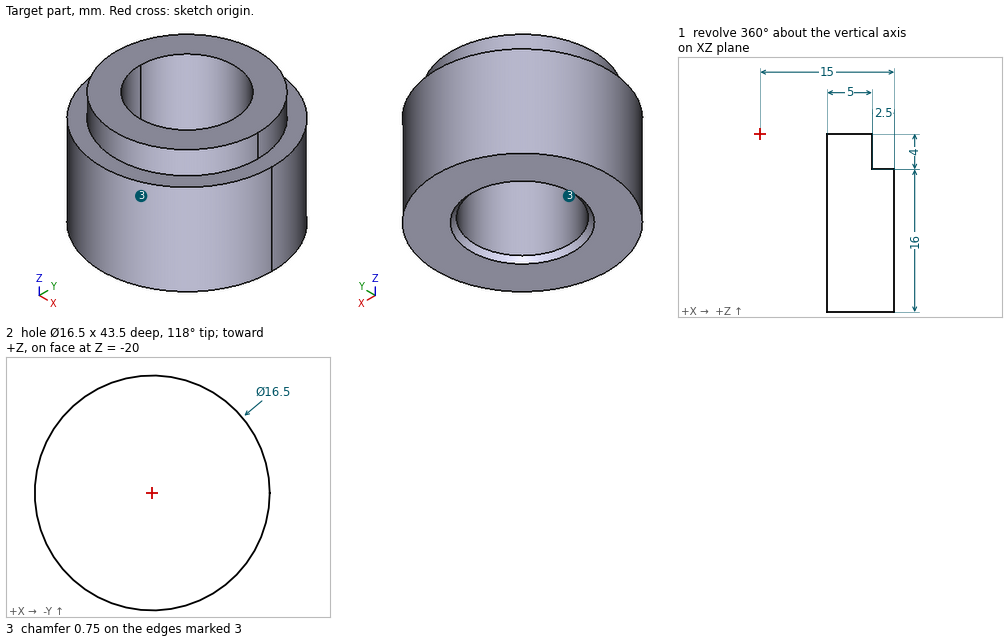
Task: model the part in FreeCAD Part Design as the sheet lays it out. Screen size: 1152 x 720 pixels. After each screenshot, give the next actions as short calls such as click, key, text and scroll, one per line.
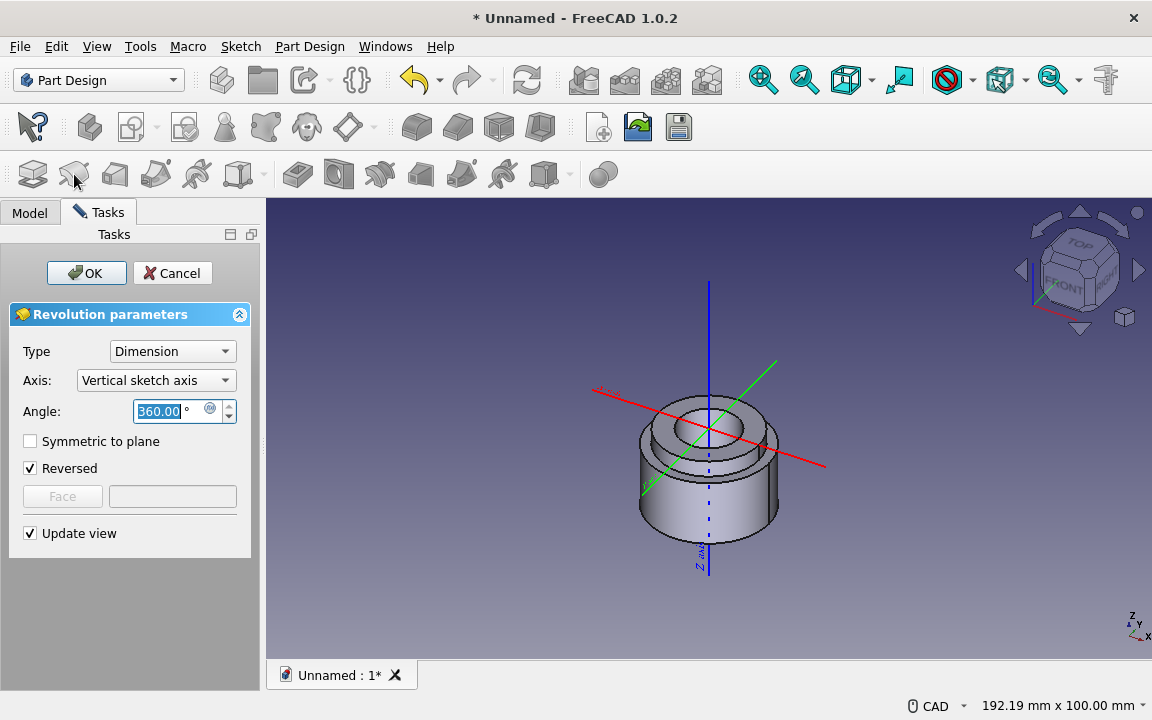
click(87, 273)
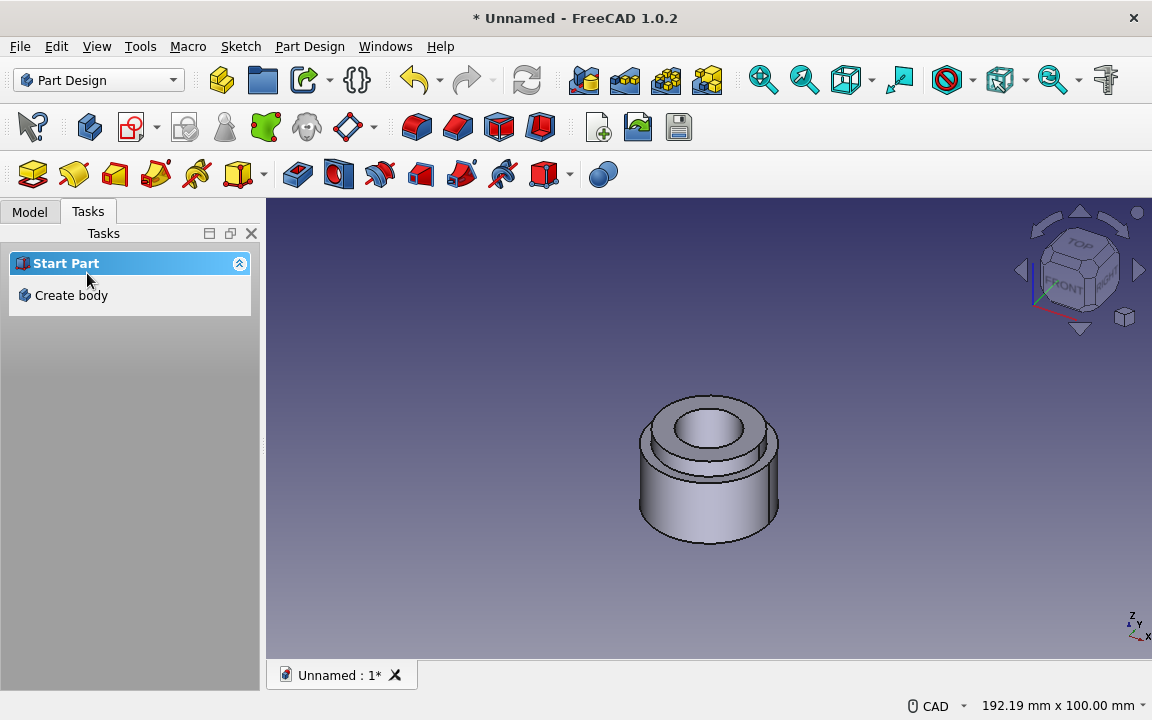
click(764, 80)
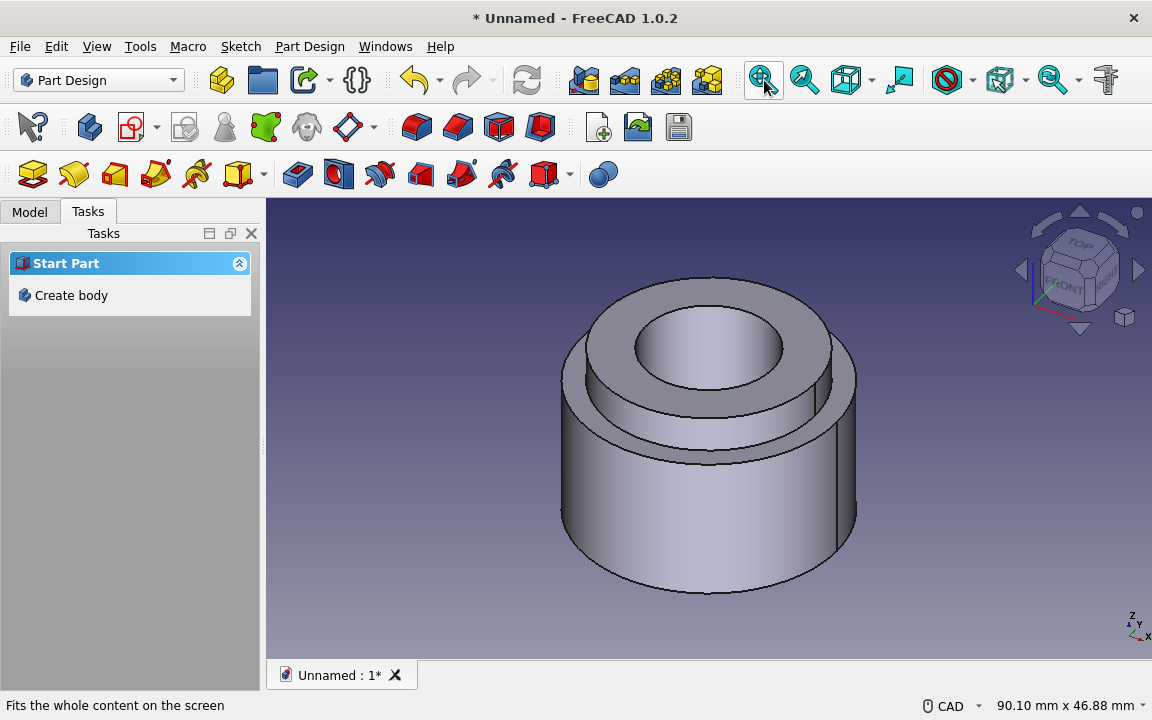
key(5)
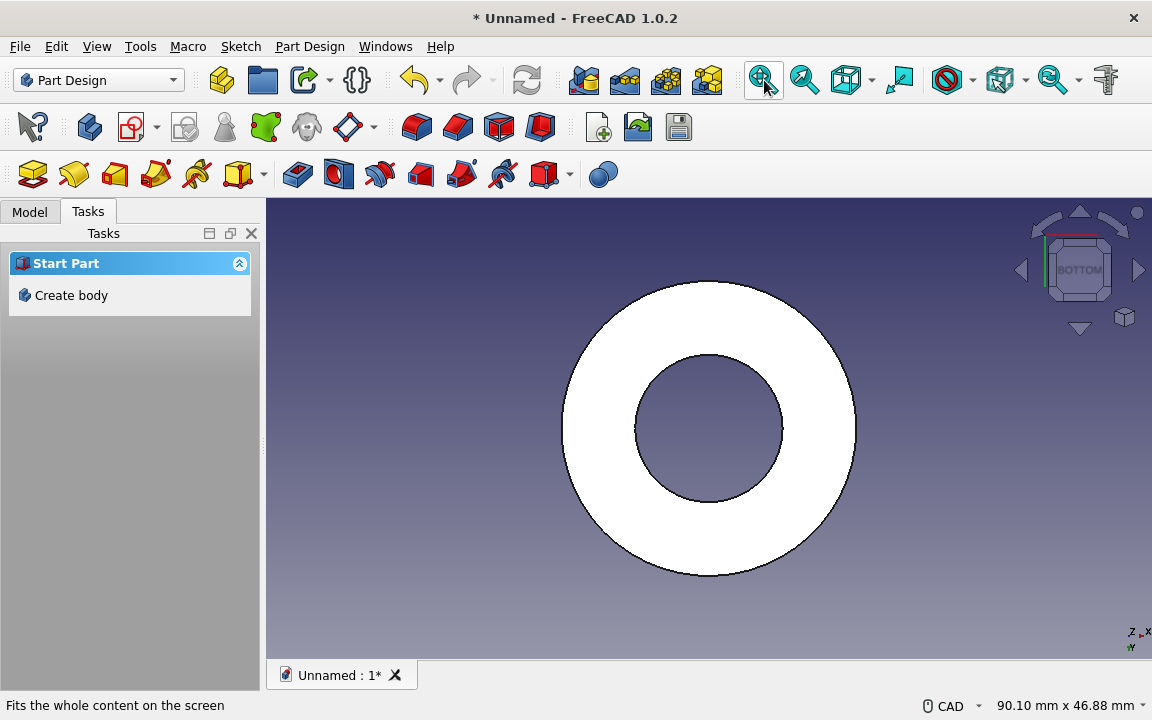
click(625, 512)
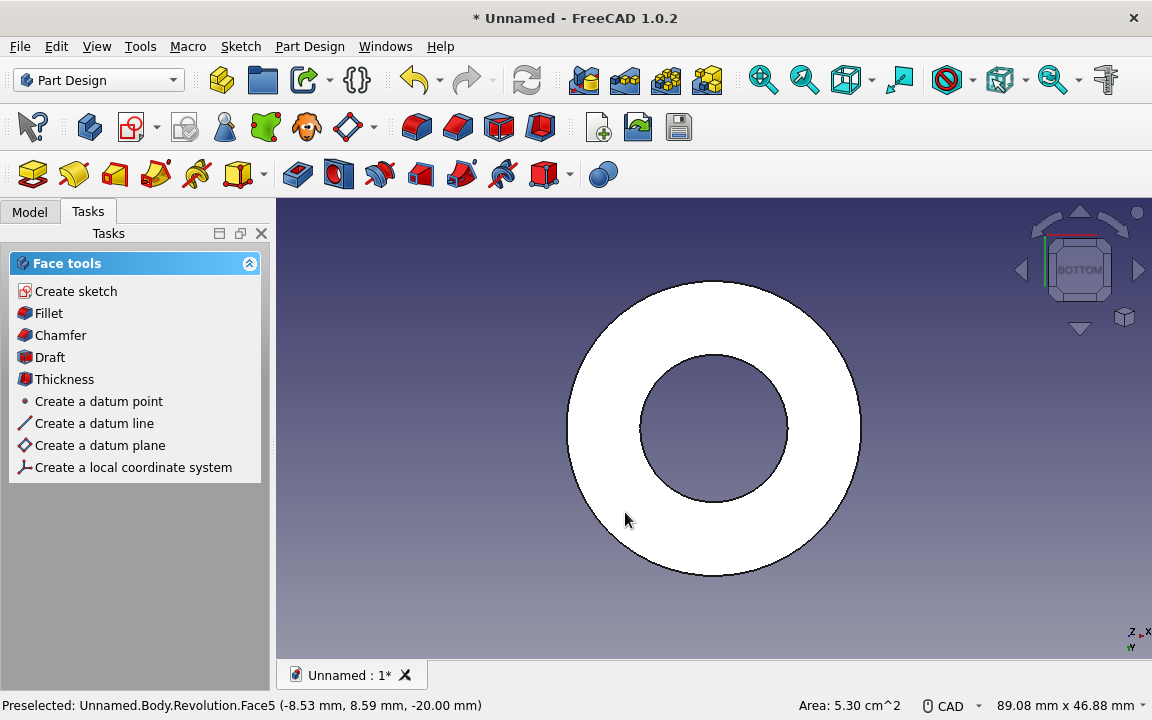
click(130, 128)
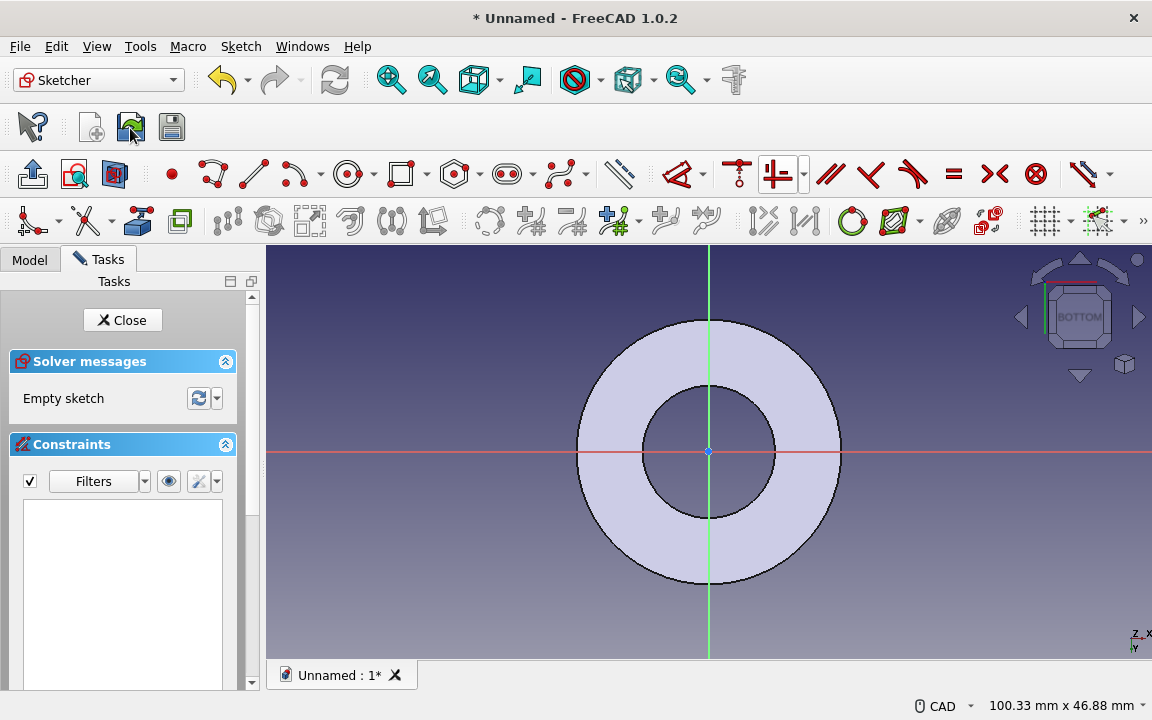
scroll(792, 452, up, 3)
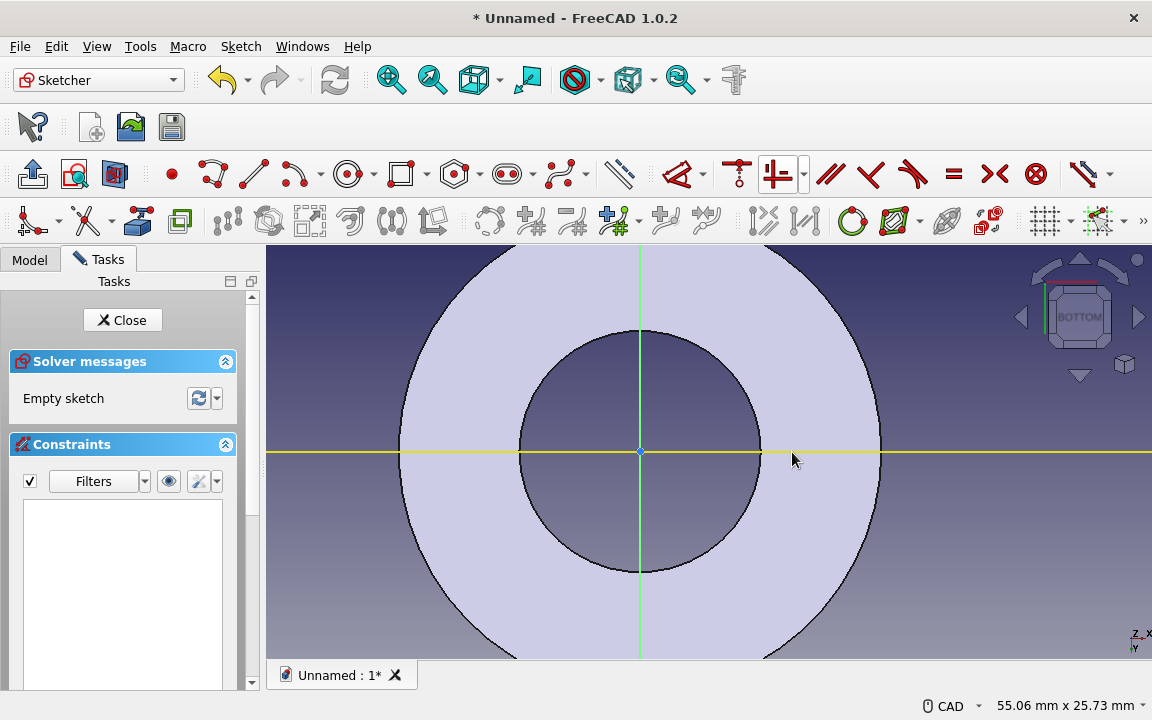
click(348, 174)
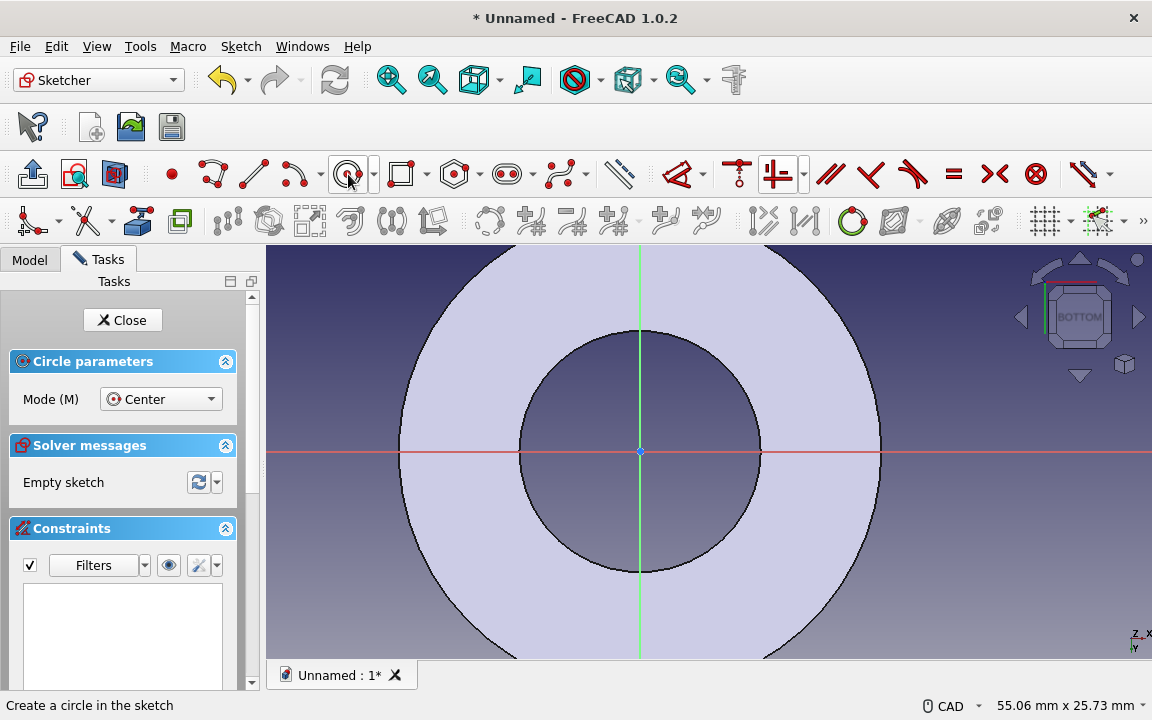
click(640, 452)
move(734, 358)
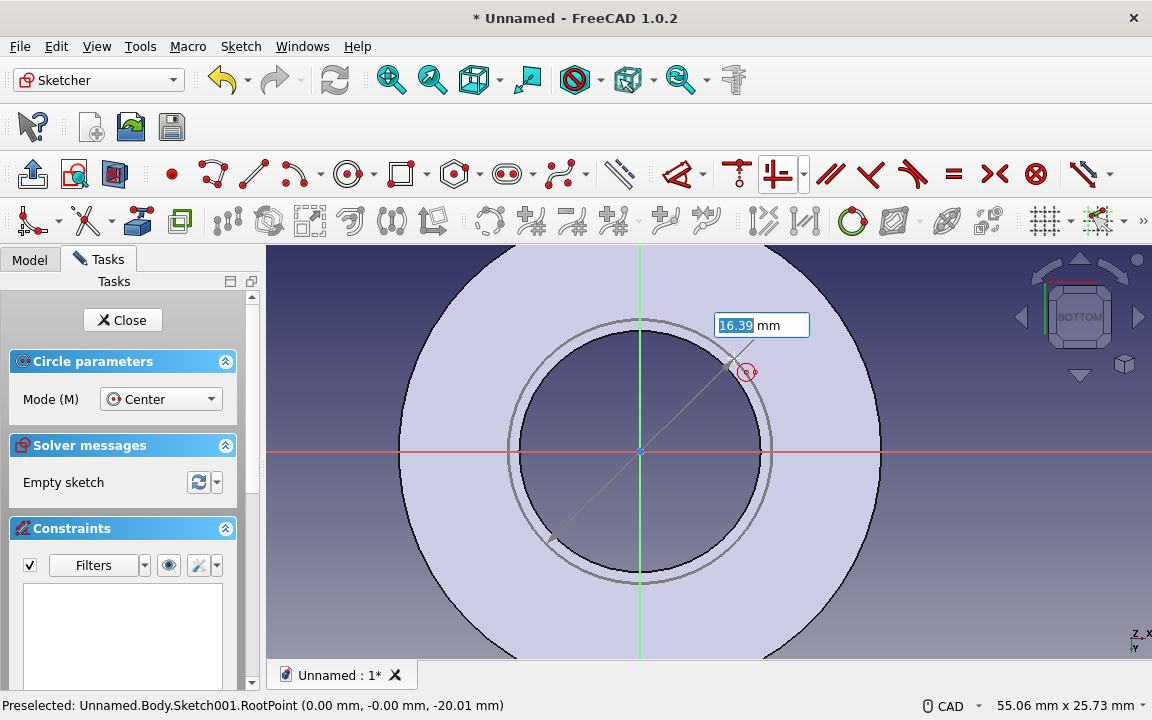
text(16.5)
key(Return)
key(Escape)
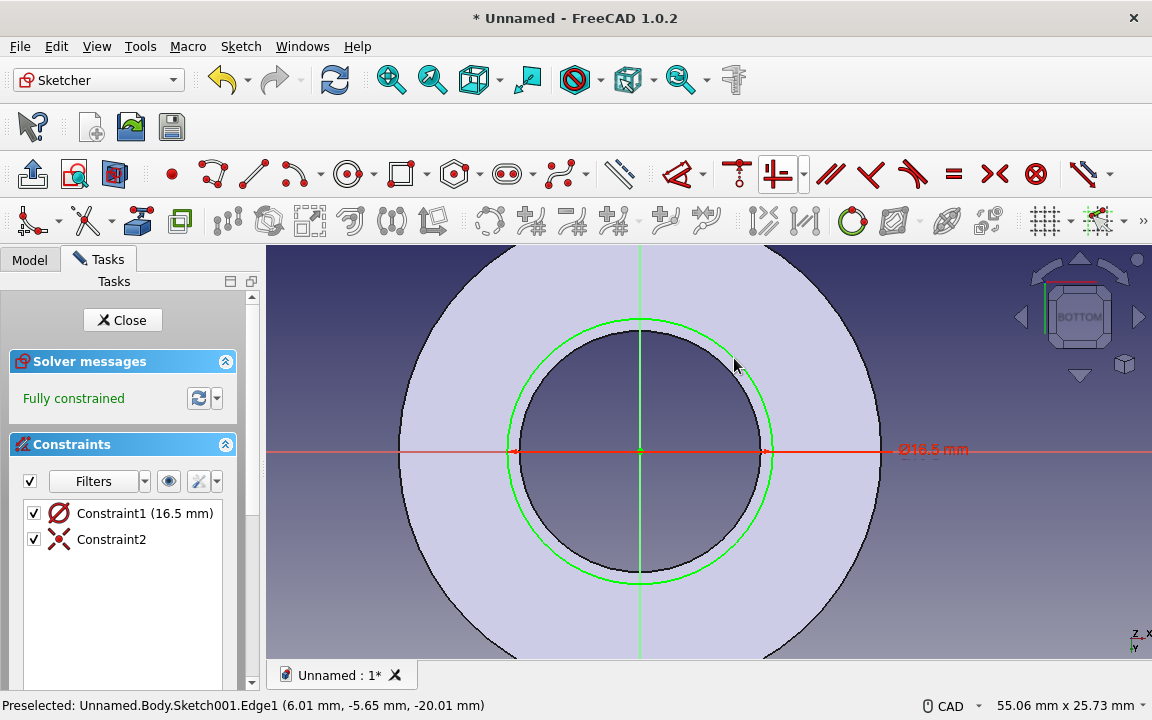
click(123, 320)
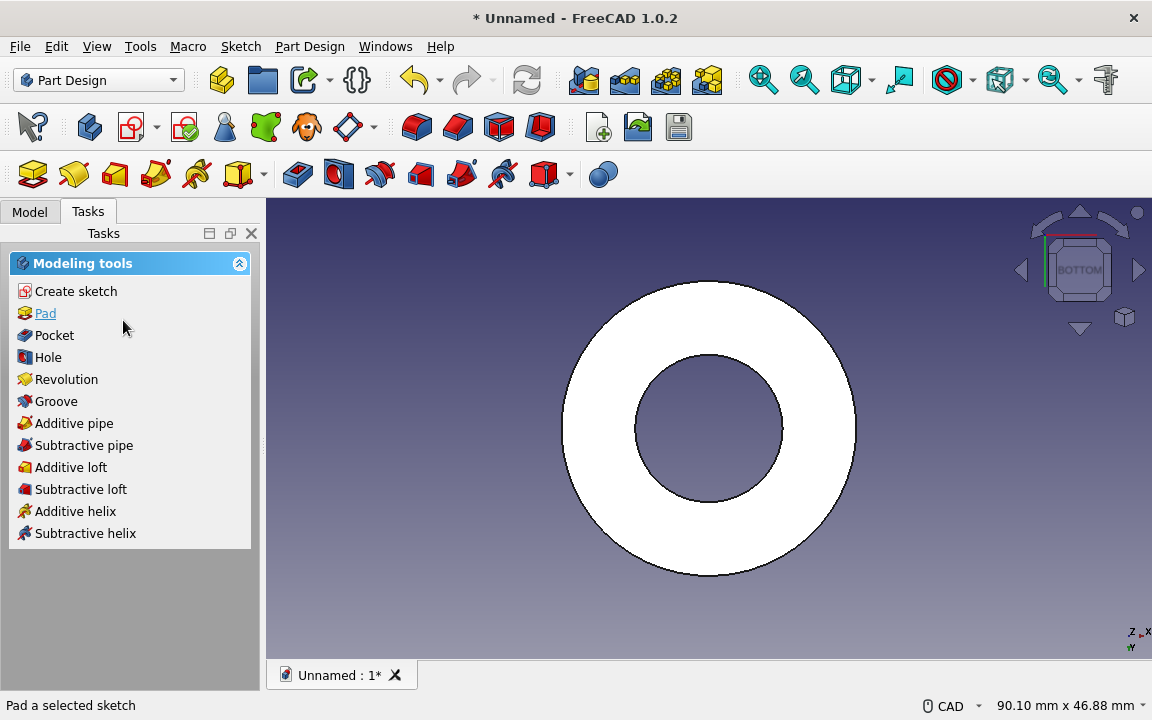
click(339, 174)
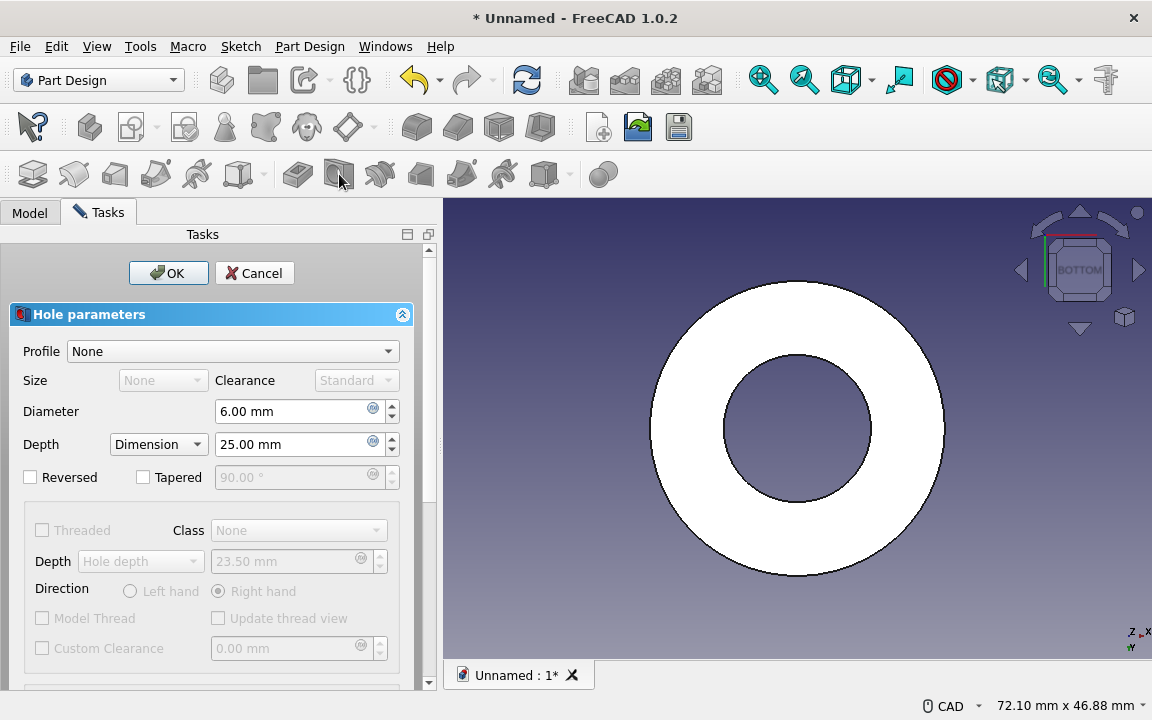
triple_click(300, 412)